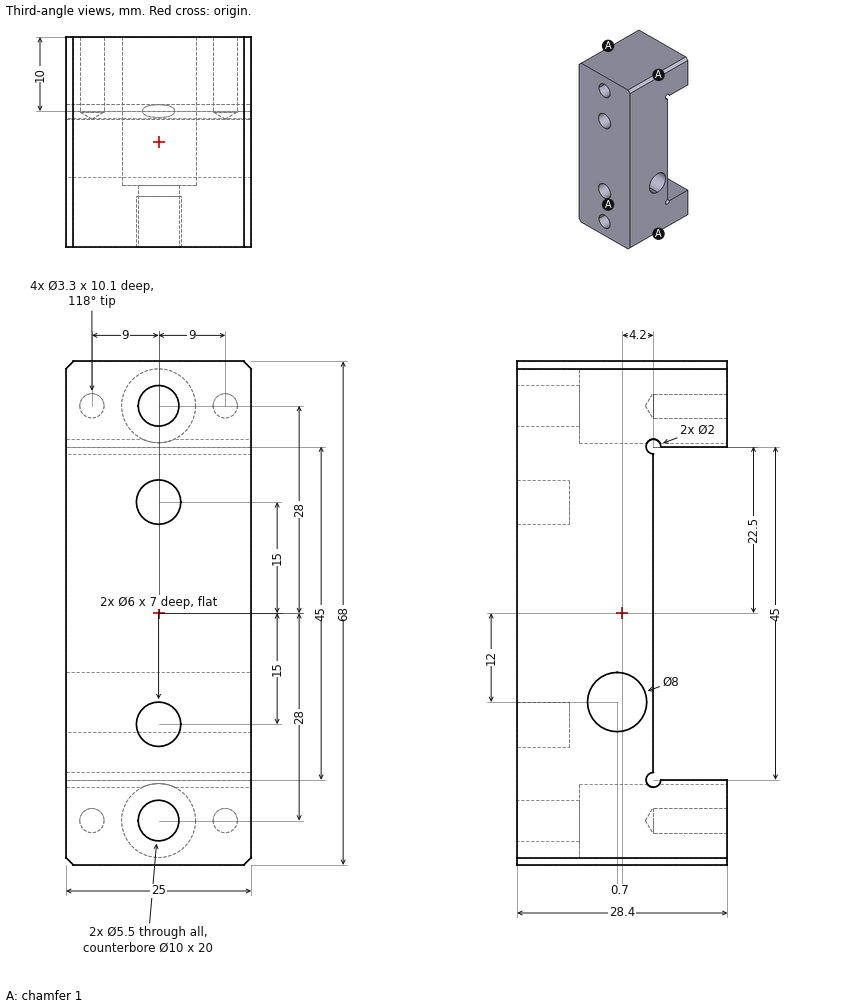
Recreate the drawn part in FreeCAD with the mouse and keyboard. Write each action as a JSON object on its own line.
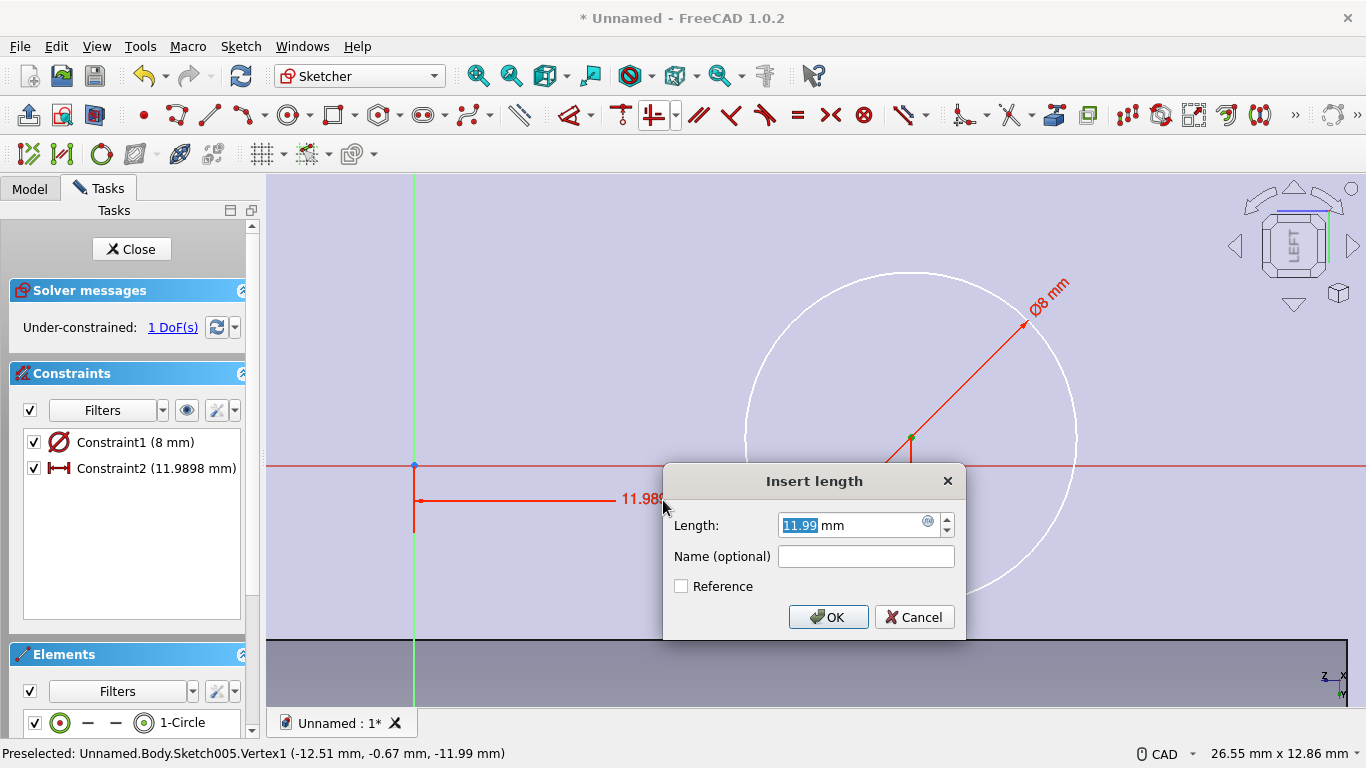
{"action": "type", "text": "12"}
{"action": "key", "text": "Return"}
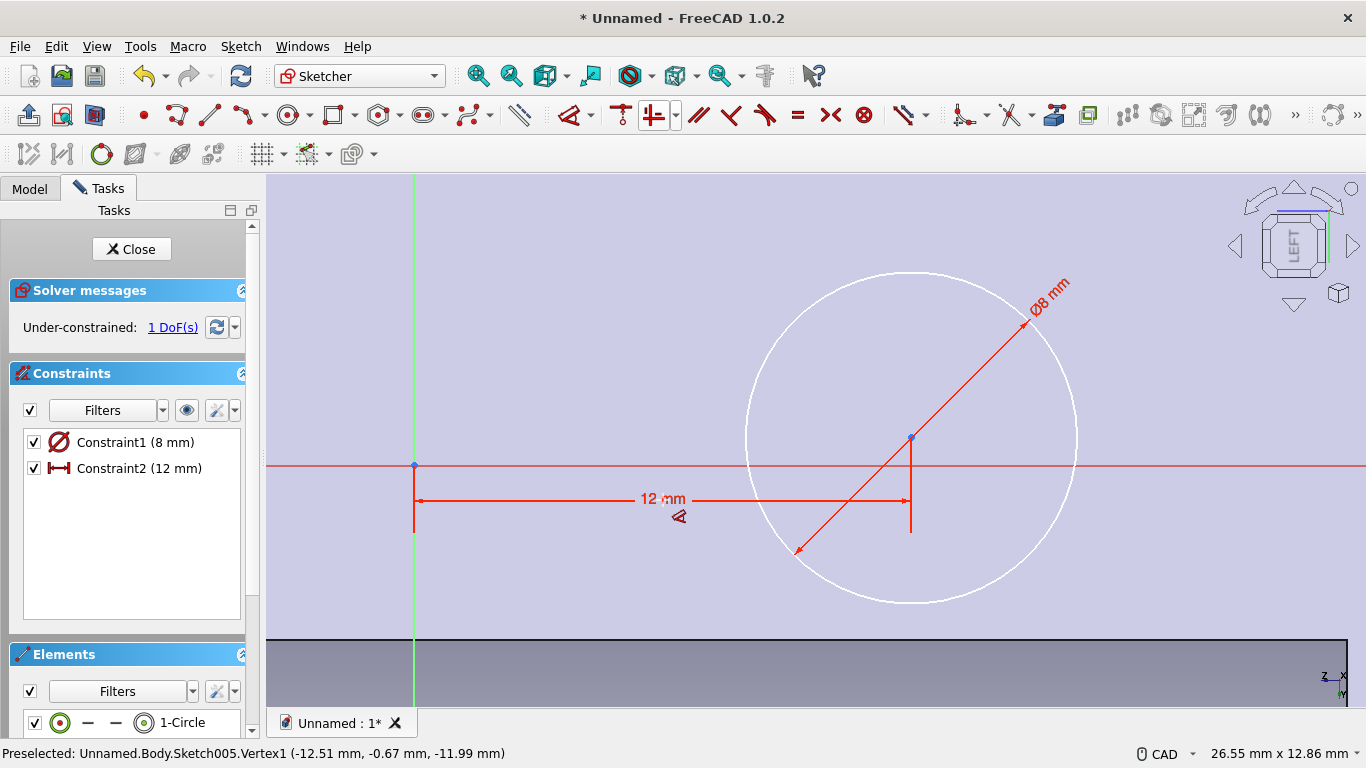
{"action": "scroll", "coordinate": [911, 438], "scroll_direction": "up", "scroll_amount": 2}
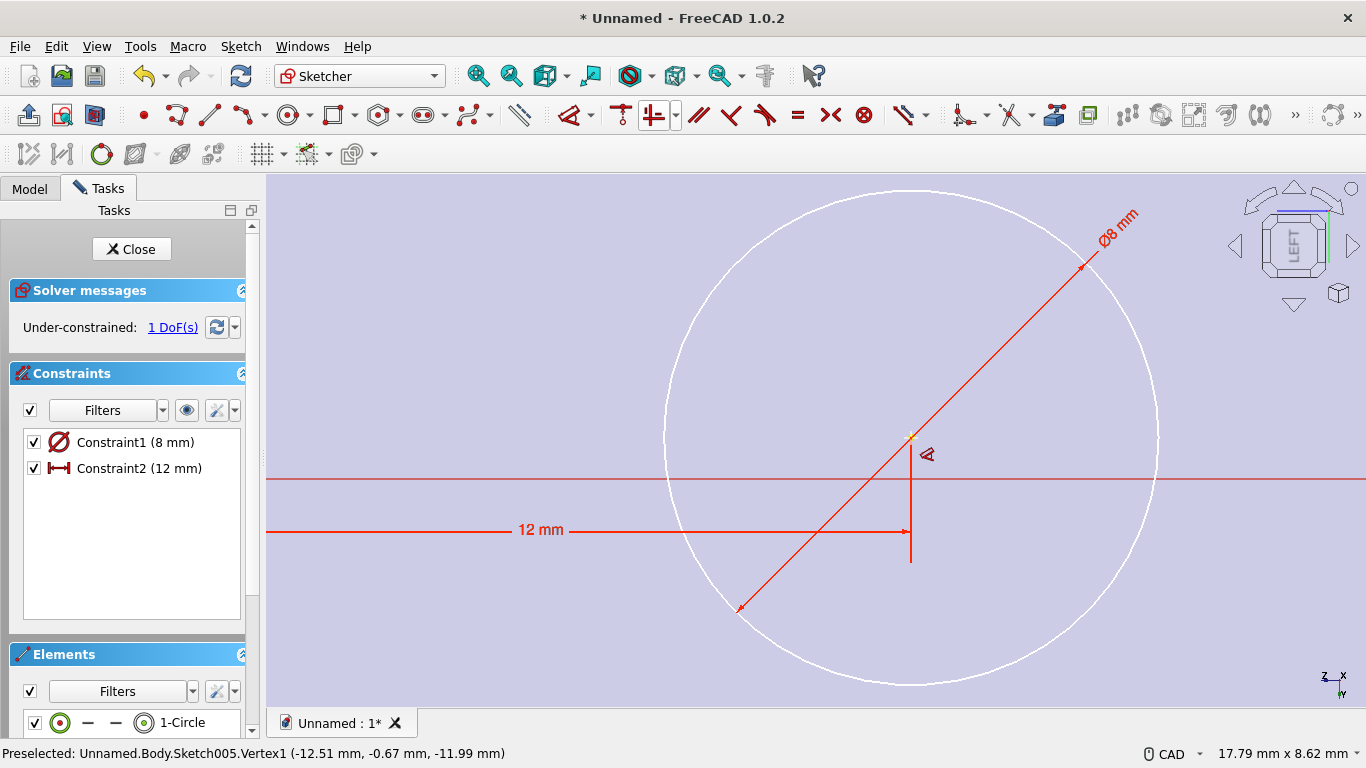
{"action": "left_click", "coordinate": [911, 438]}
{"action": "left_click", "coordinate": [945, 458]}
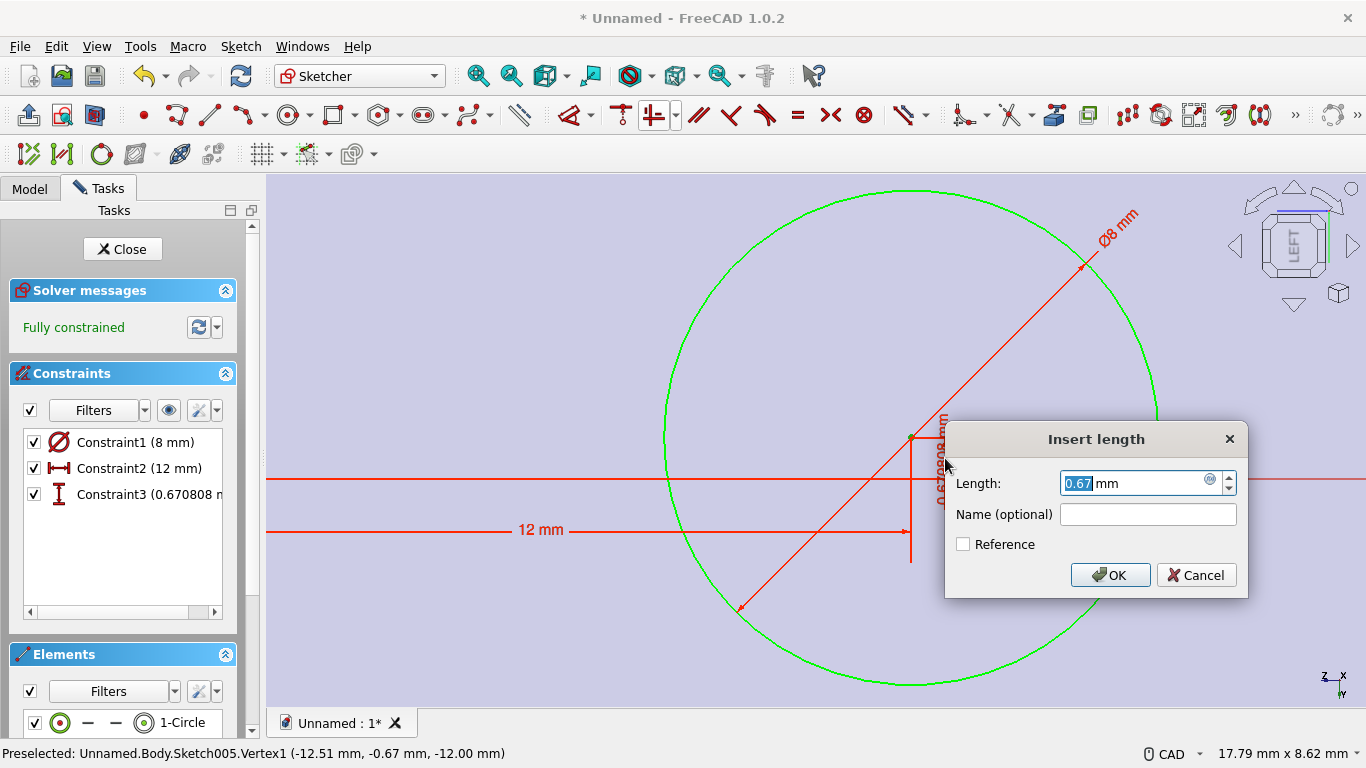
{"action": "type", "text": "0.7"}
{"action": "key", "text": "Return"}
{"action": "key", "text": "Escape"}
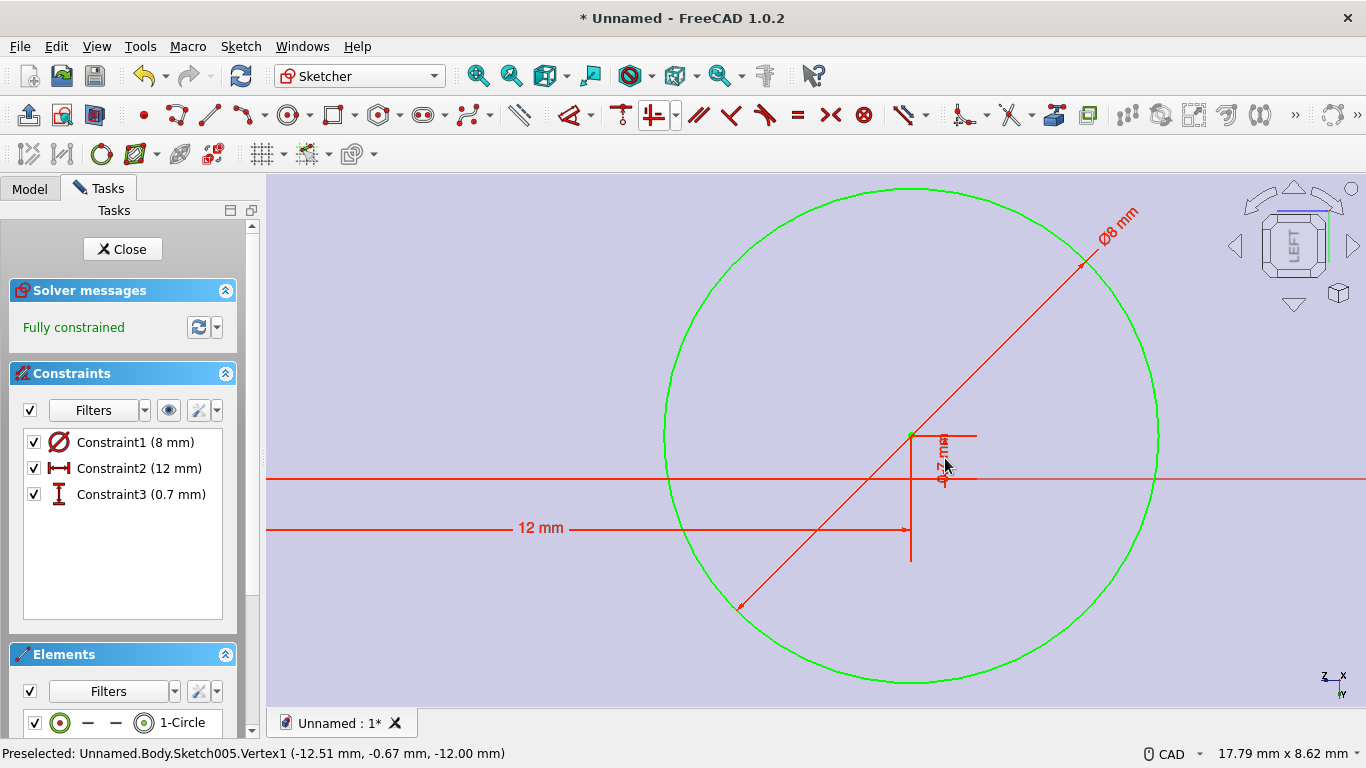
{"action": "left_click", "coordinate": [123, 249]}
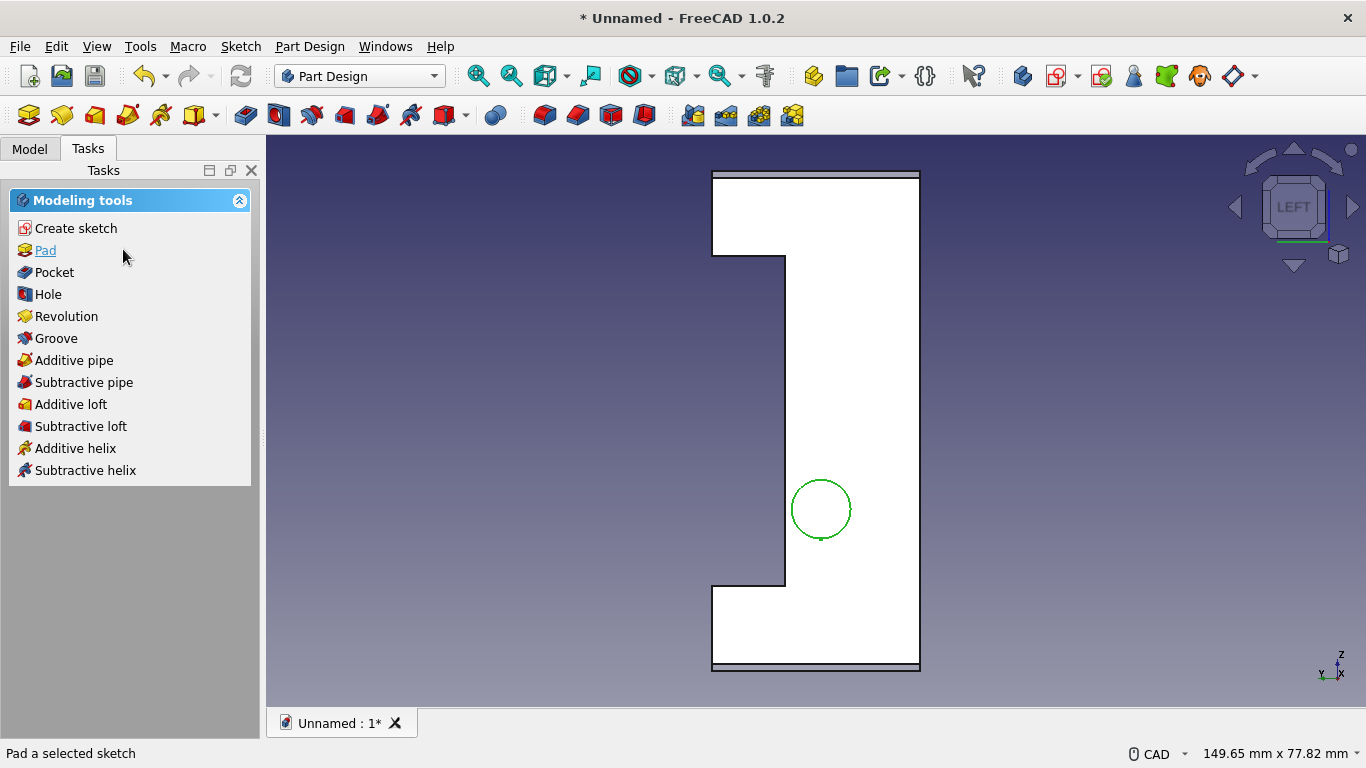
{"action": "left_click", "coordinate": [246, 116]}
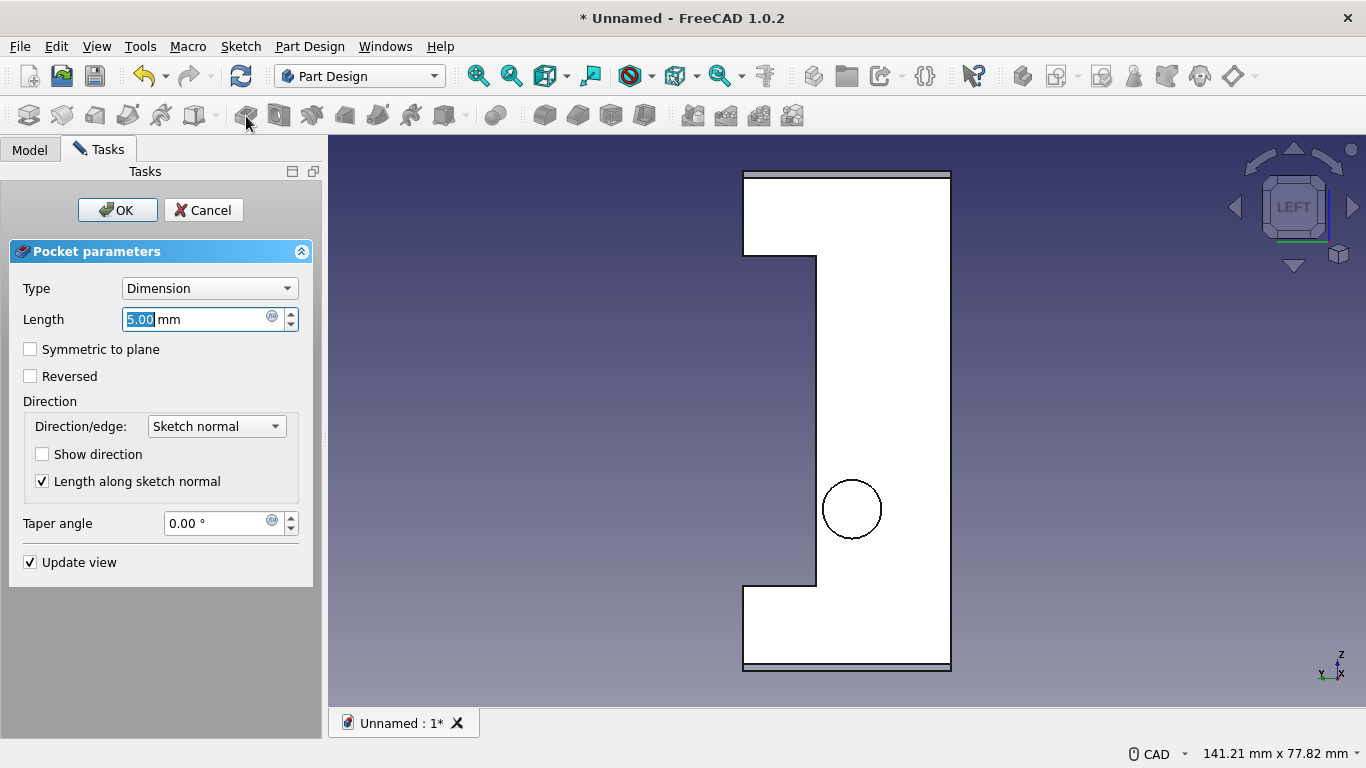
{"action": "left_click", "coordinate": [210, 288]}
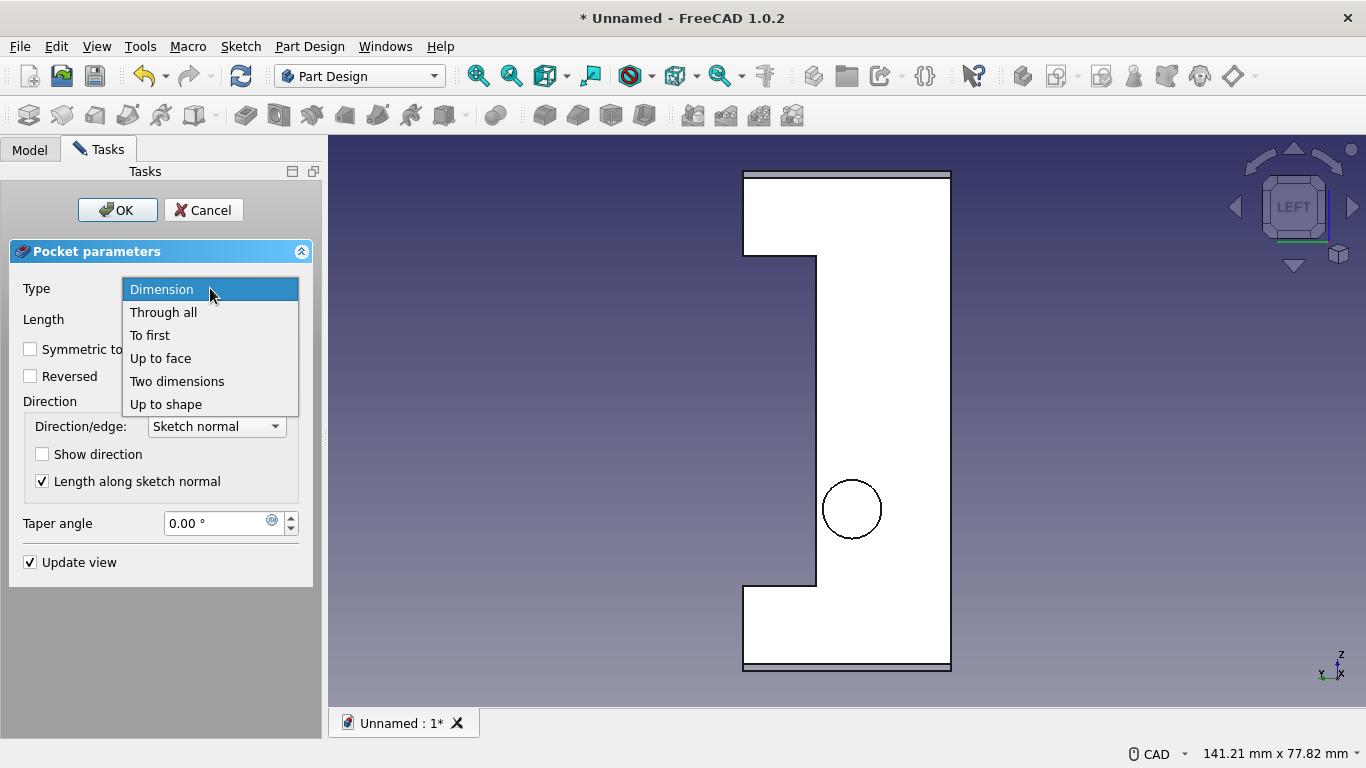
{"action": "left_click", "coordinate": [208, 312]}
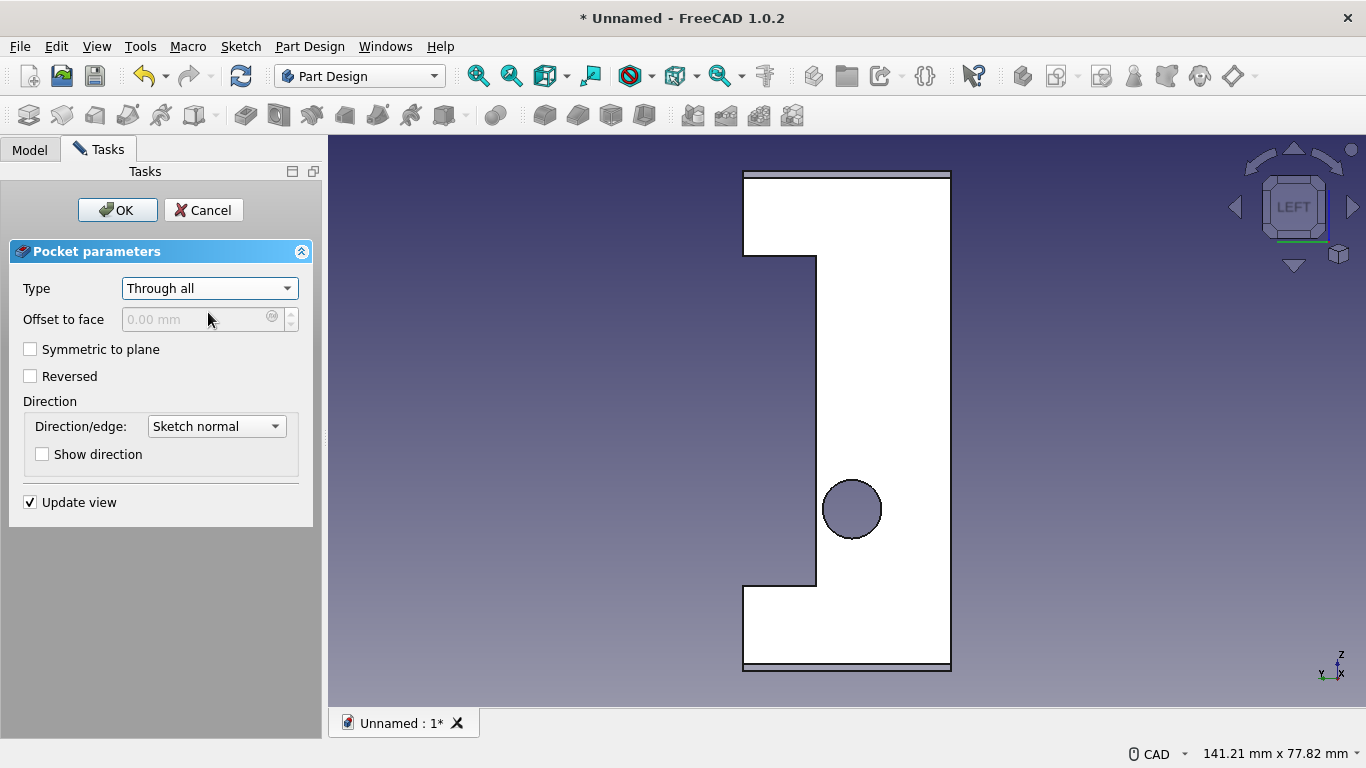
{"action": "left_click", "coordinate": [118, 210]}